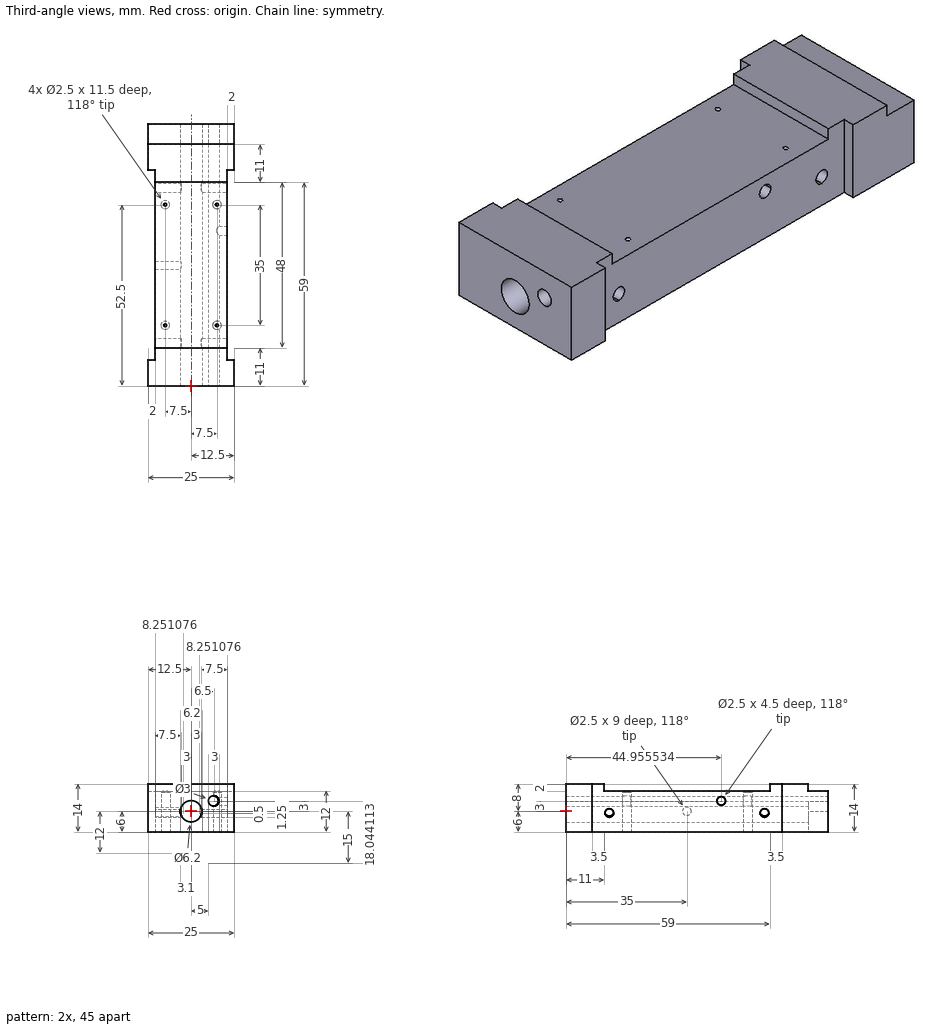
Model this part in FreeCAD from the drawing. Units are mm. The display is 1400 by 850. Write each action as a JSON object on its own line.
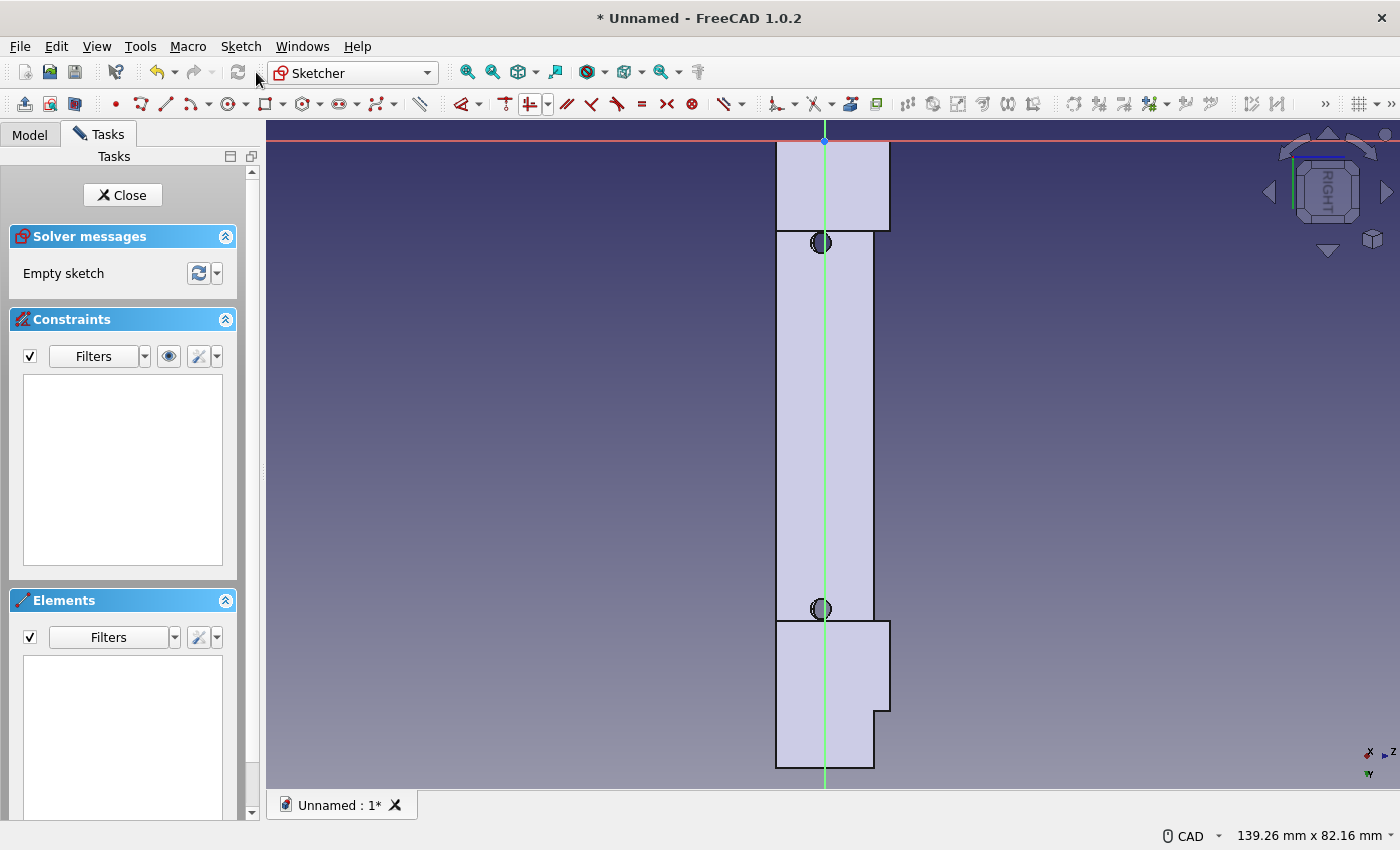
{"action": "scroll", "coordinate": [455, 721], "scroll_direction": "down", "scroll_amount": 1}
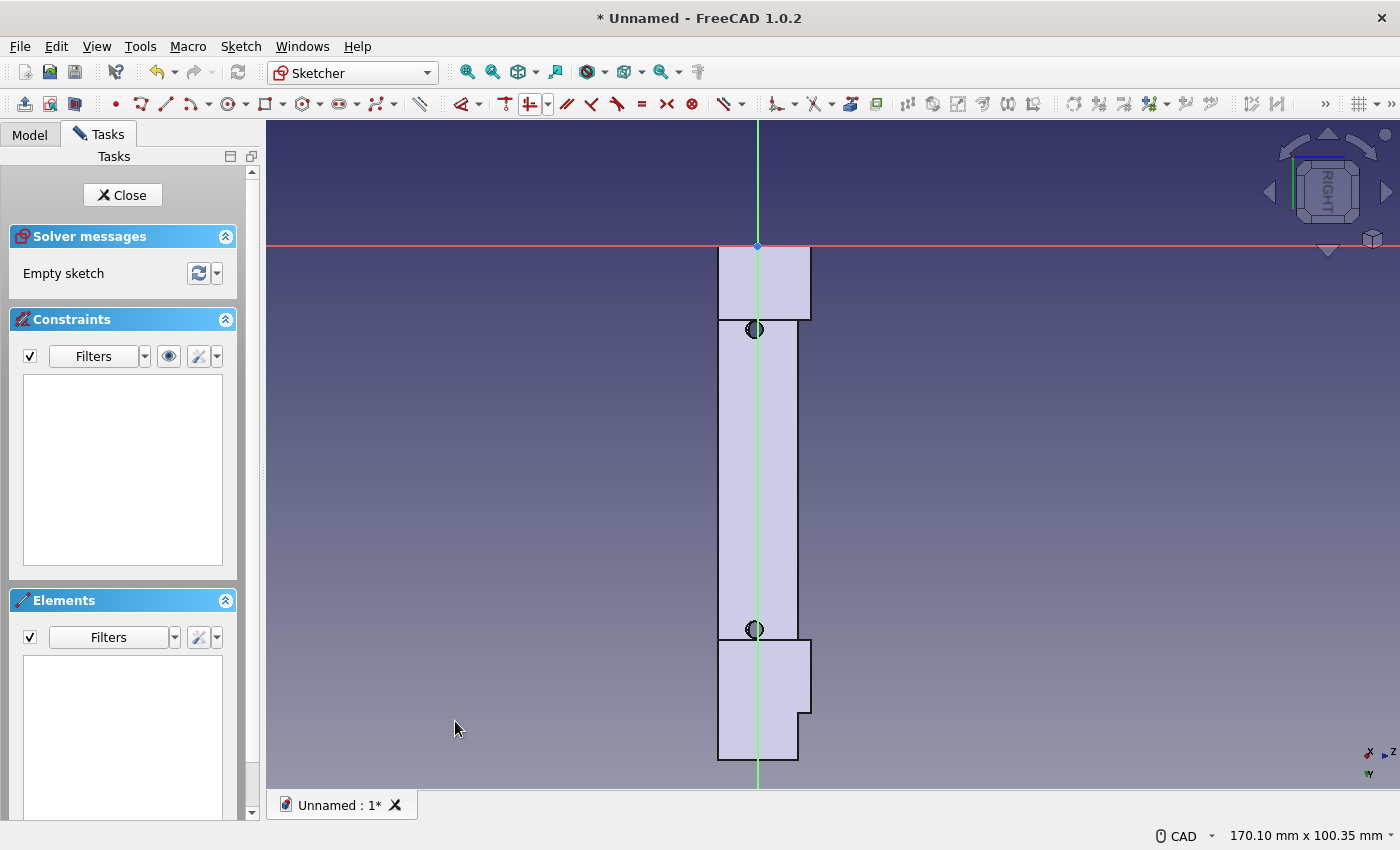
{"action": "left_click", "coordinate": [264, 104]}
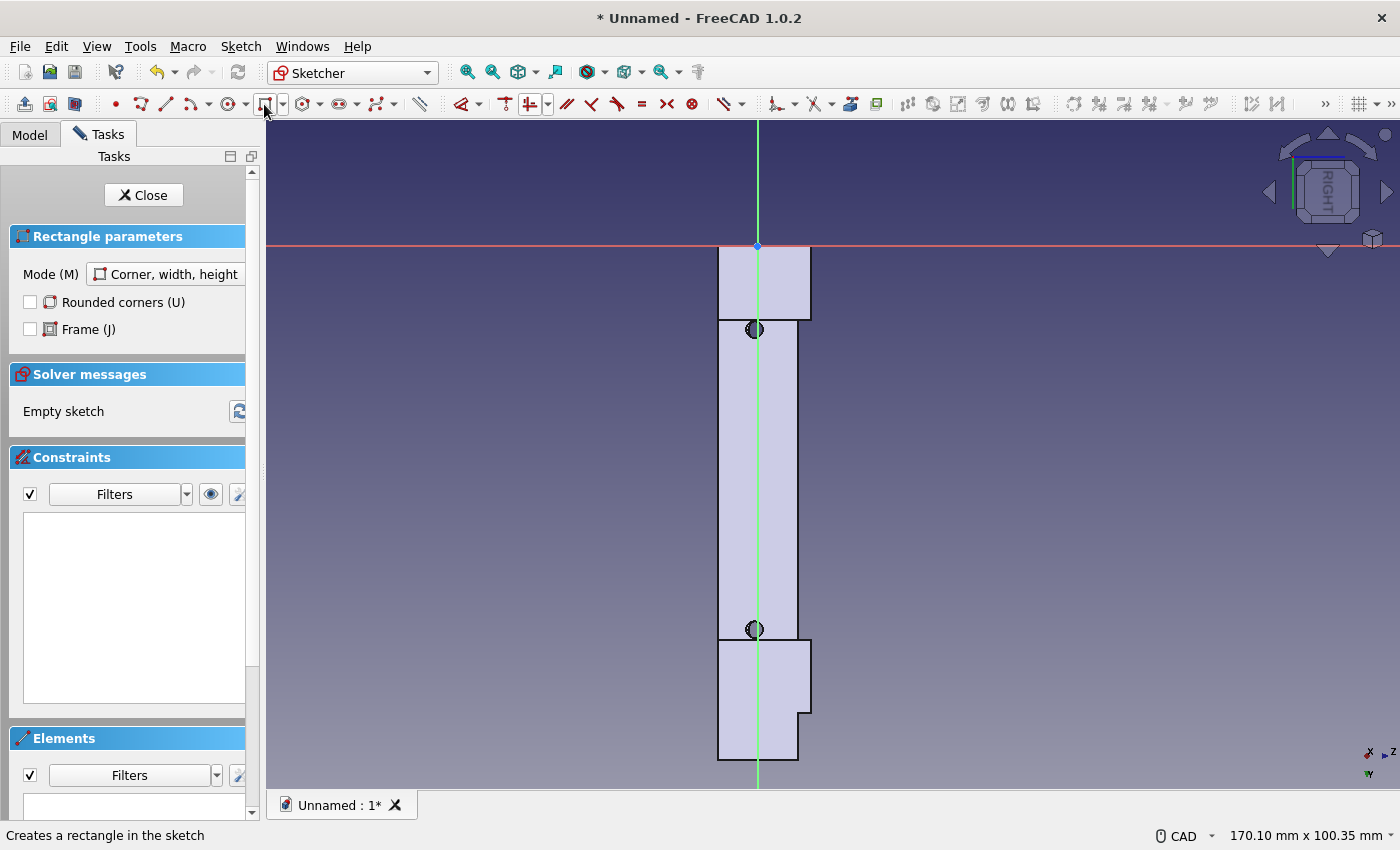
{"action": "left_click", "coordinate": [718, 640]}
{"action": "left_click", "coordinate": [811, 663]}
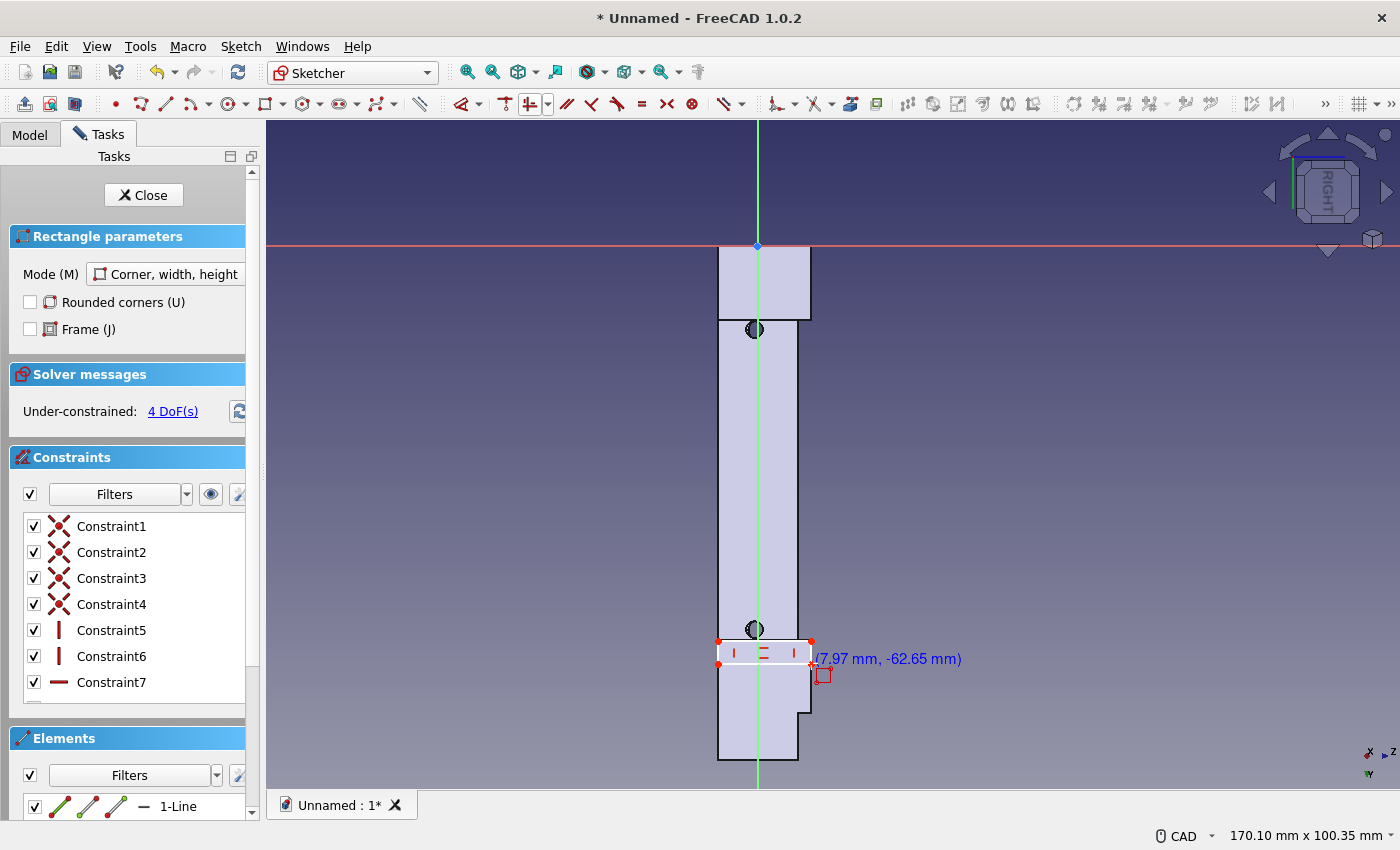
{"action": "left_click", "coordinate": [718, 296]}
{"action": "left_click", "coordinate": [811, 320]}
{"action": "key", "text": "Escape"}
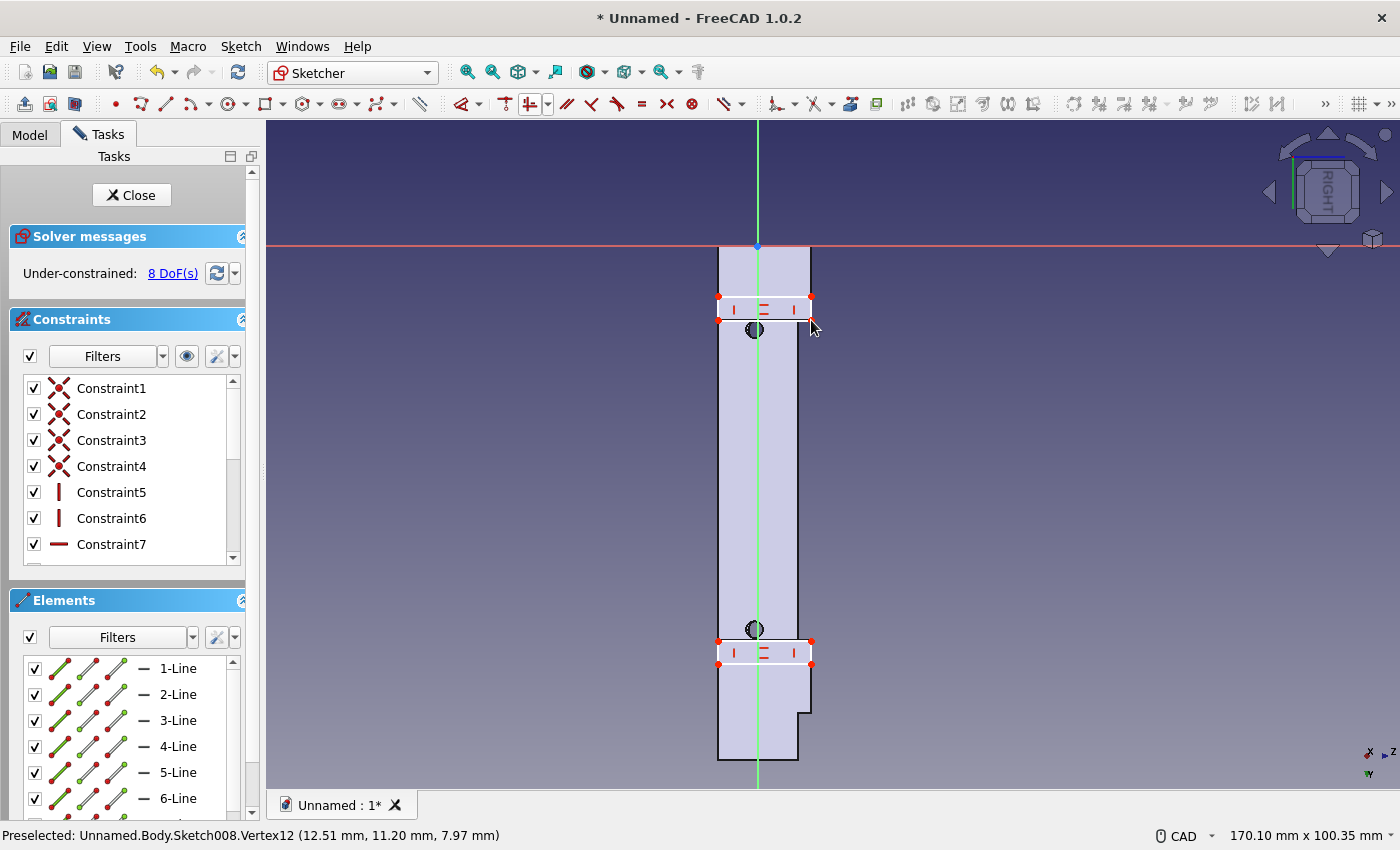
{"action": "left_click", "coordinate": [460, 104]}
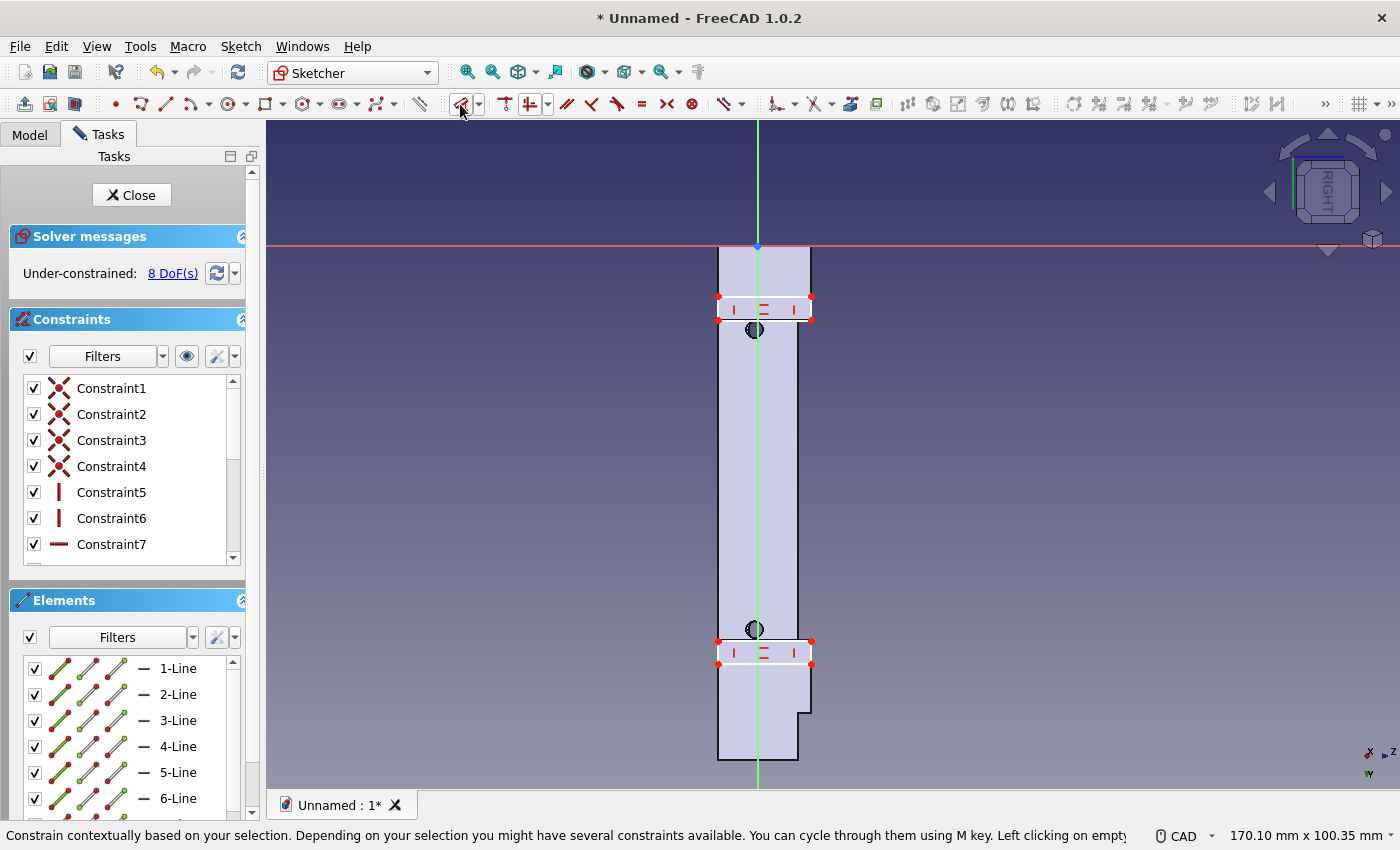
{"action": "left_click", "coordinate": [746, 664]}
{"action": "left_click", "coordinate": [743, 698]}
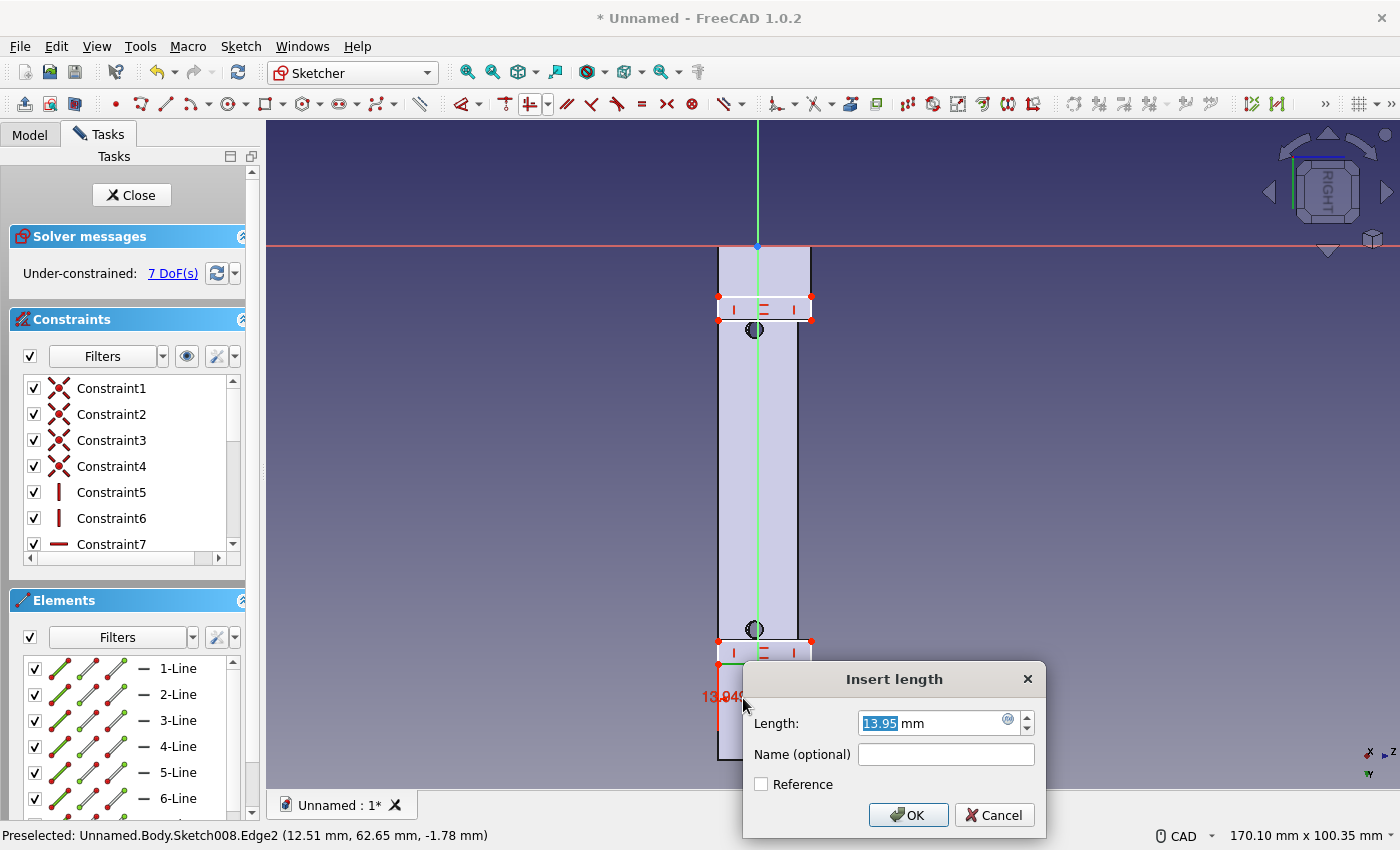
{"action": "type", "text": "14"}
{"action": "key", "text": "Return"}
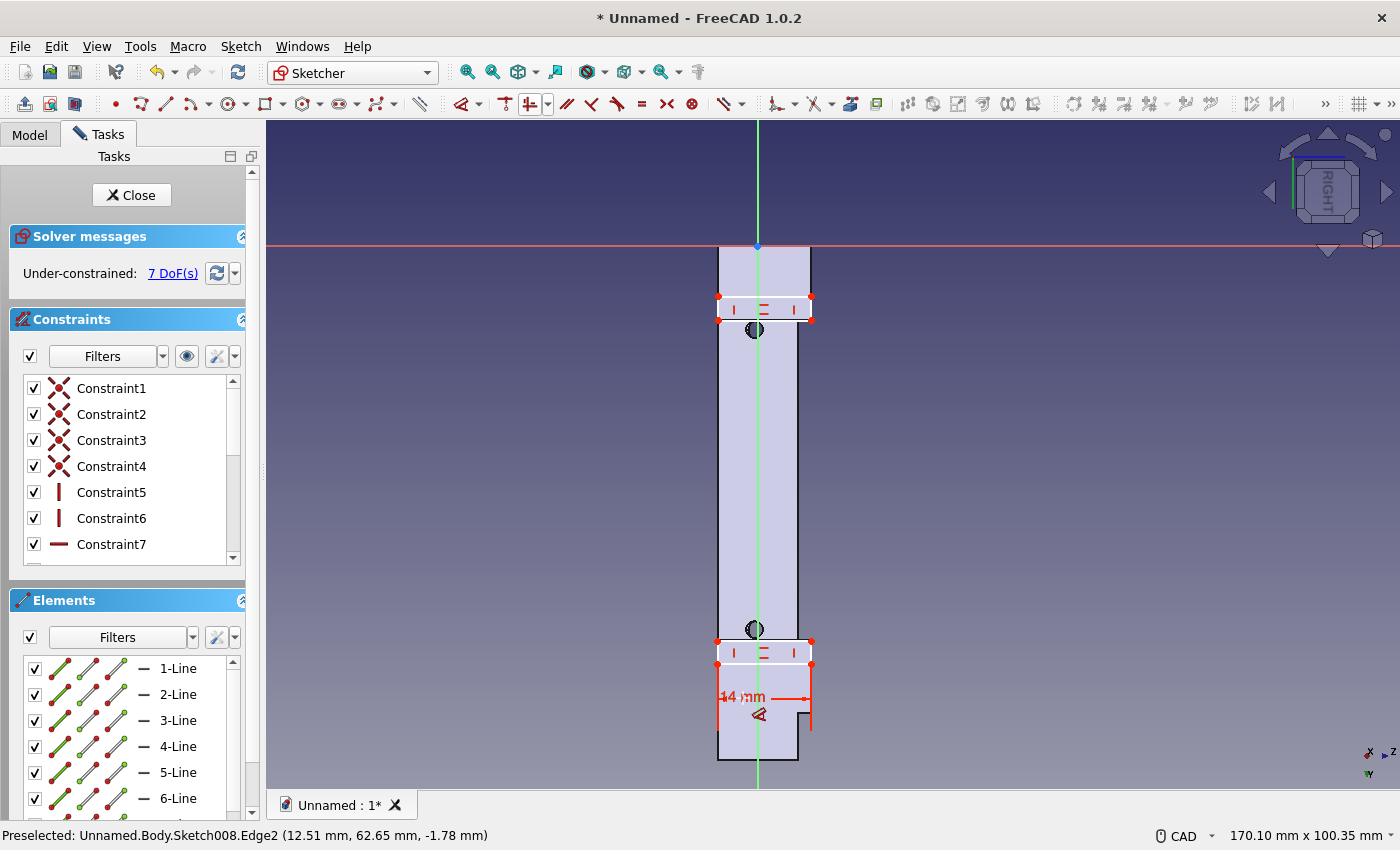
{"action": "left_click", "coordinate": [746, 321]}
{"action": "left_click", "coordinate": [743, 355]}